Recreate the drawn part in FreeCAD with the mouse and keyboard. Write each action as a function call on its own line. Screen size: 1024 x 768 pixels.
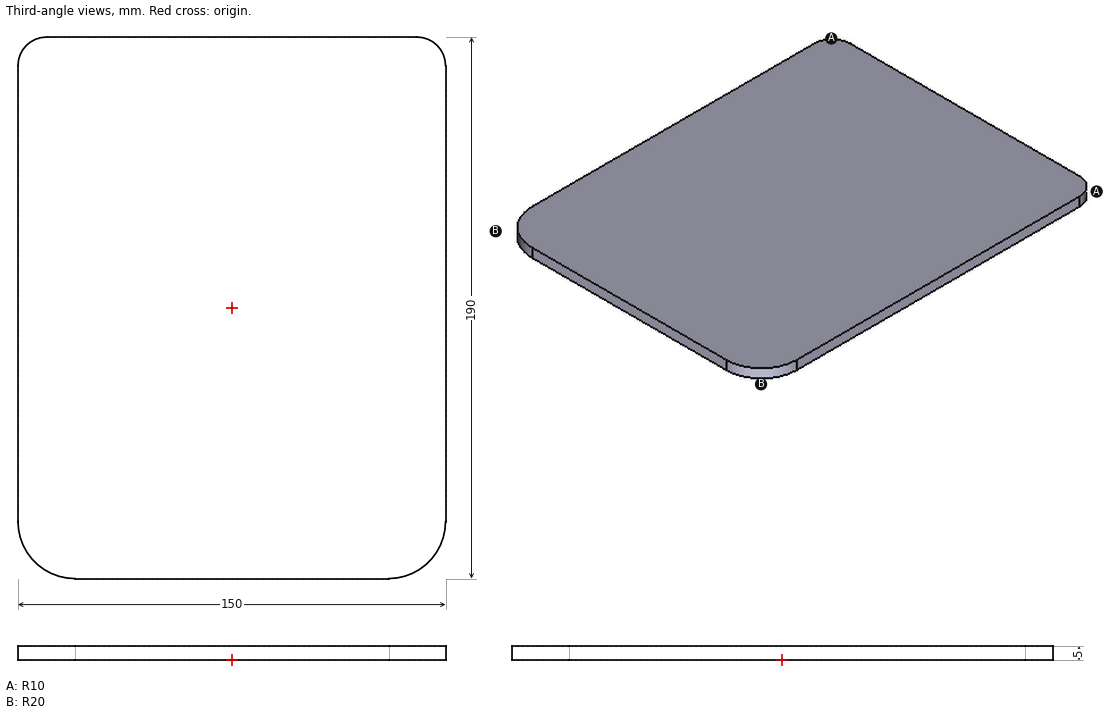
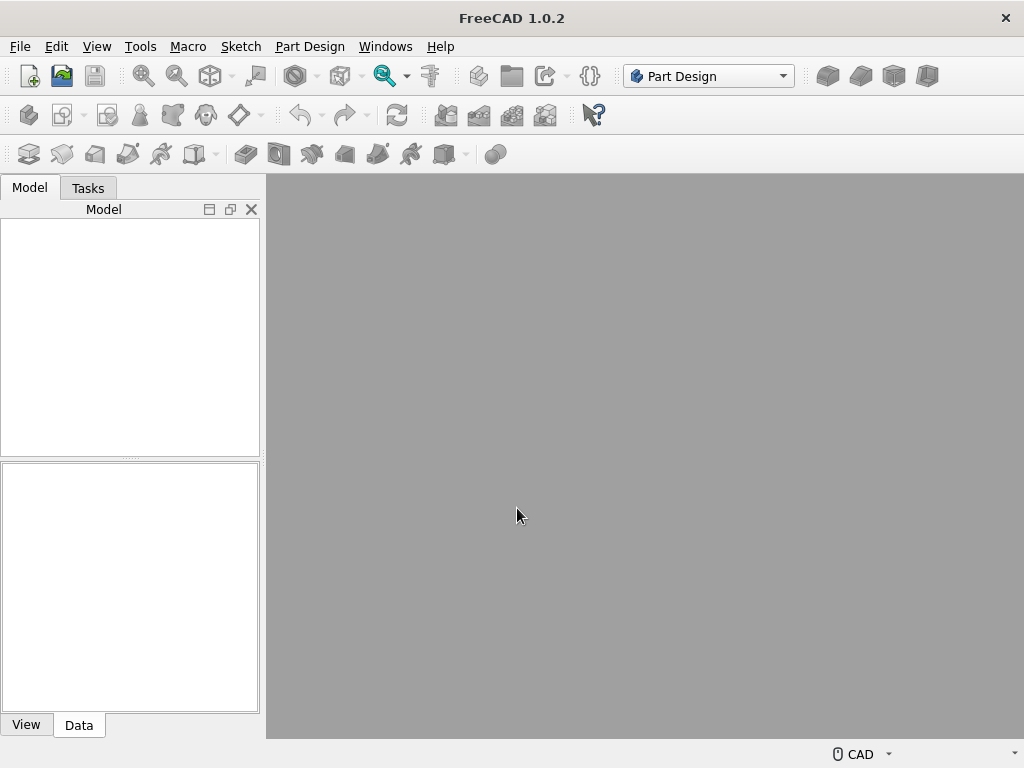
click(29, 76)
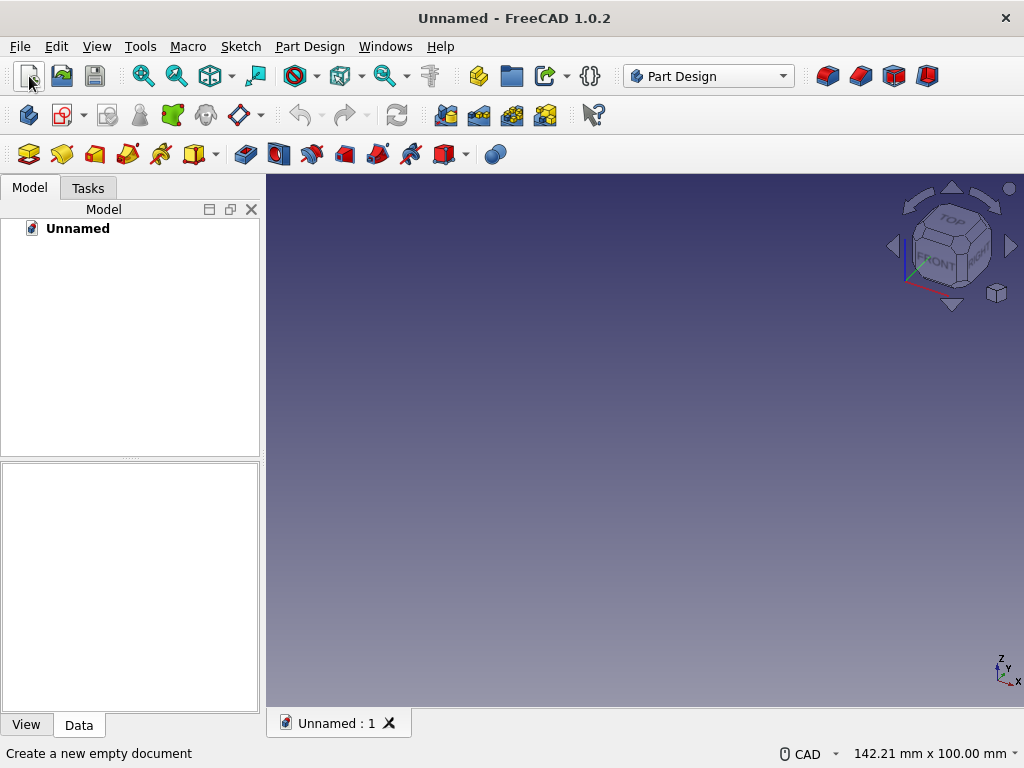
click(62, 116)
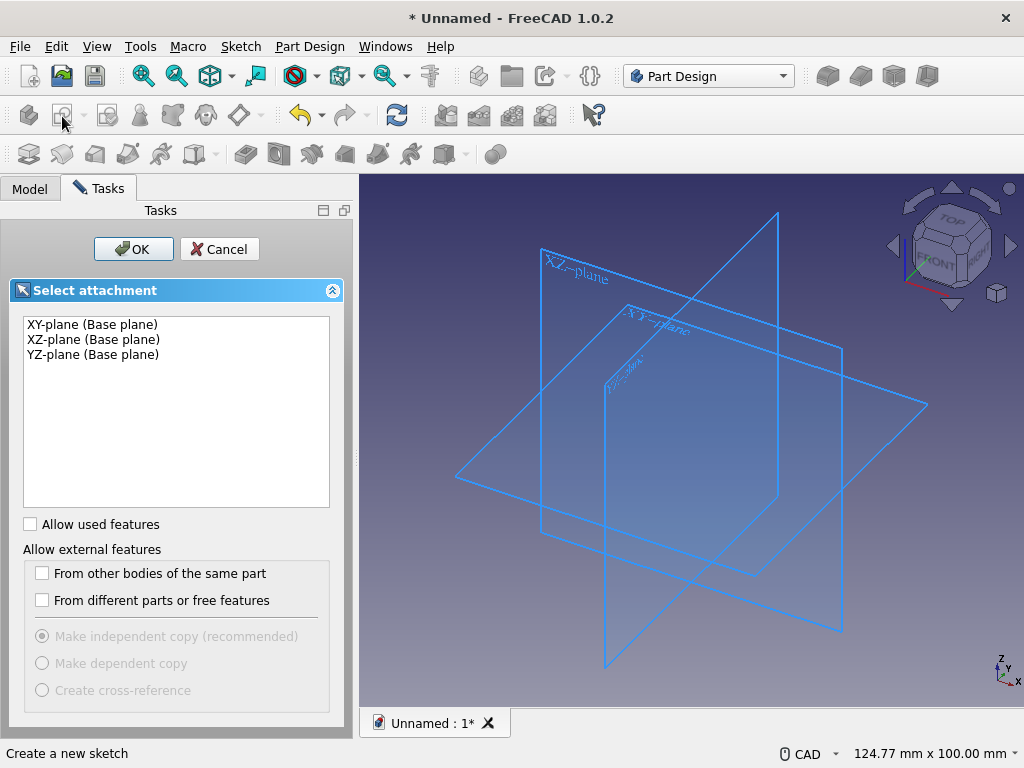
click(84, 324)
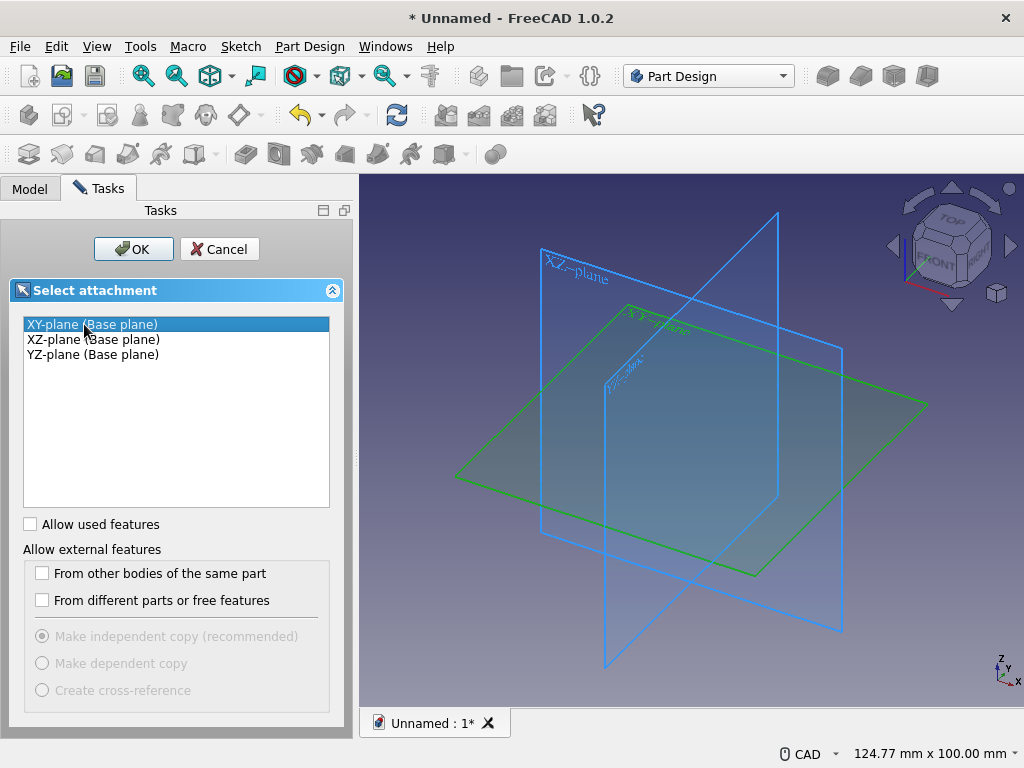
click(134, 249)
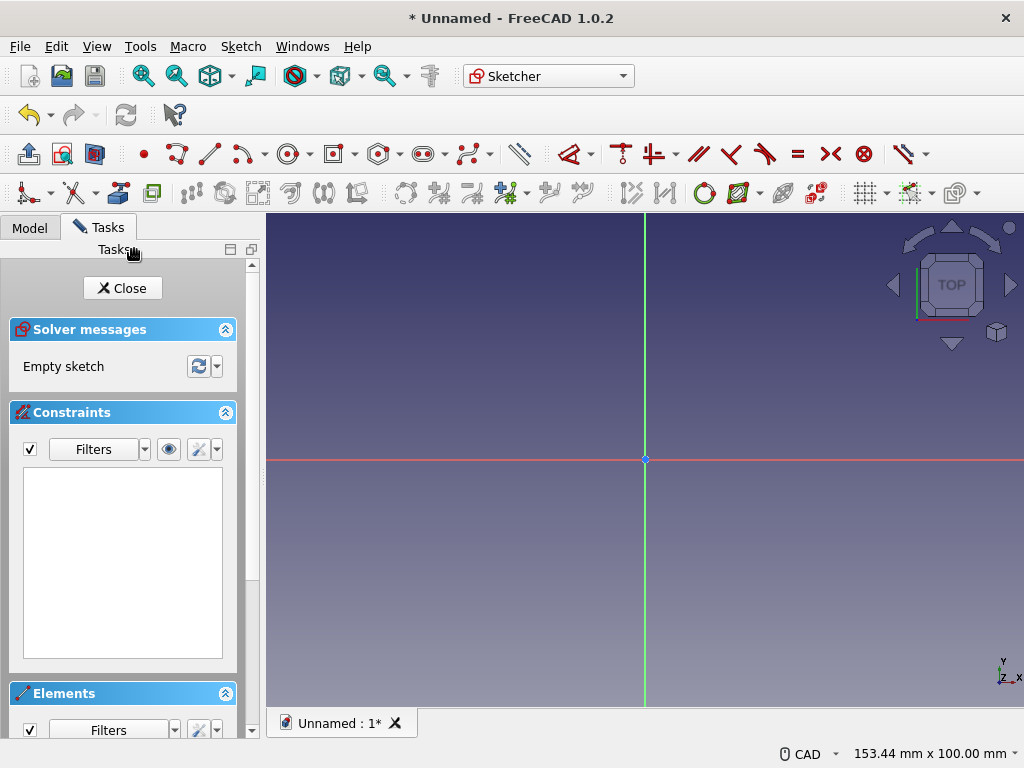
scroll(547, 460, down, 6)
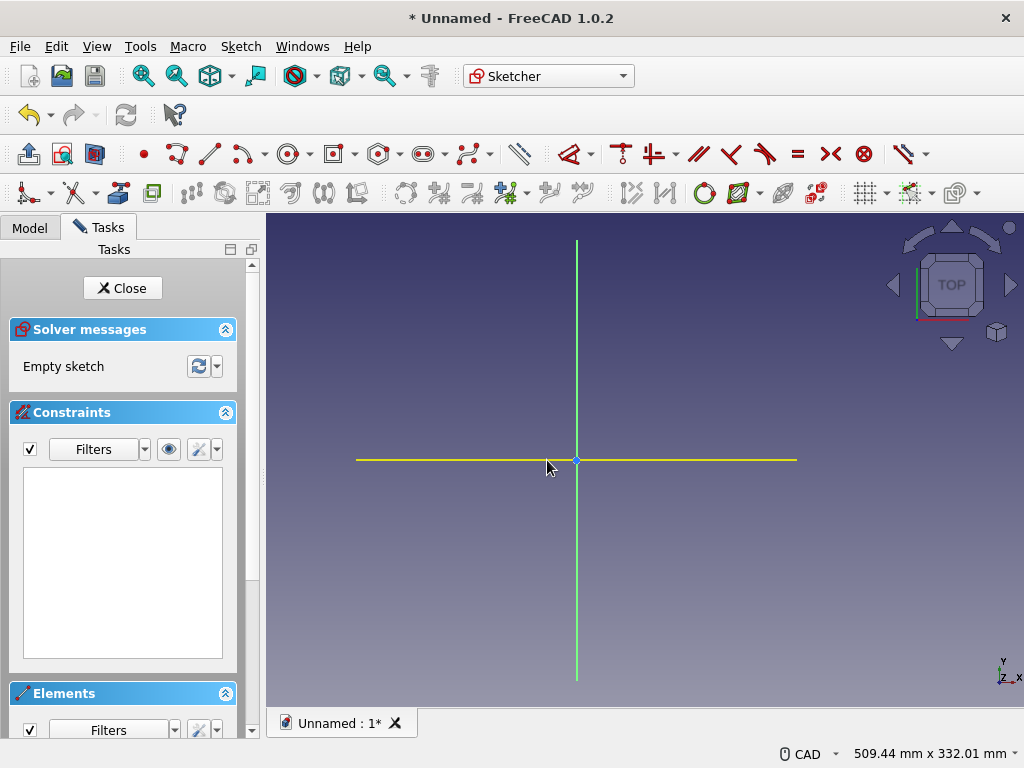
click(332, 154)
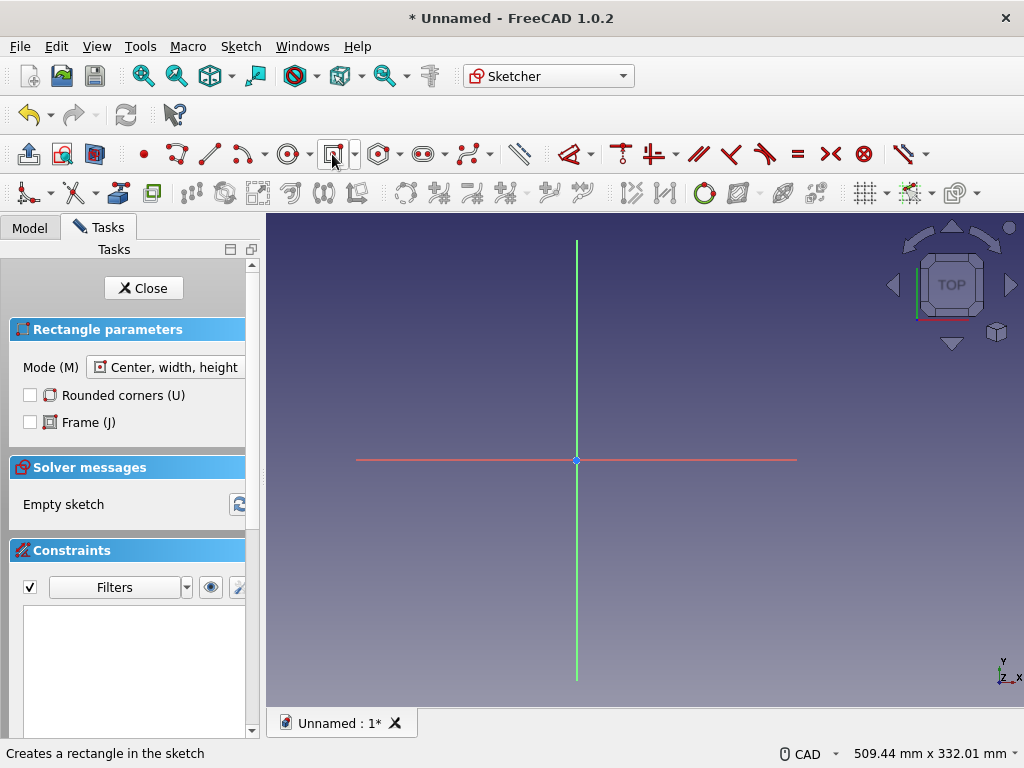
click(577, 460)
click(688, 319)
key(Escape)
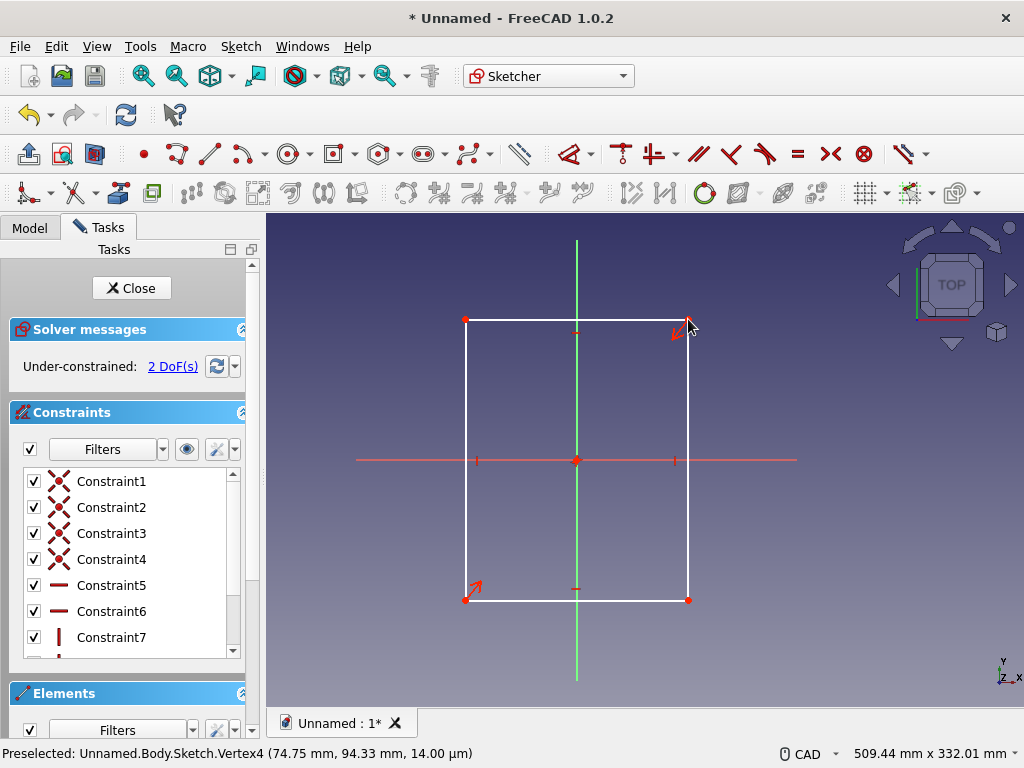
click(568, 154)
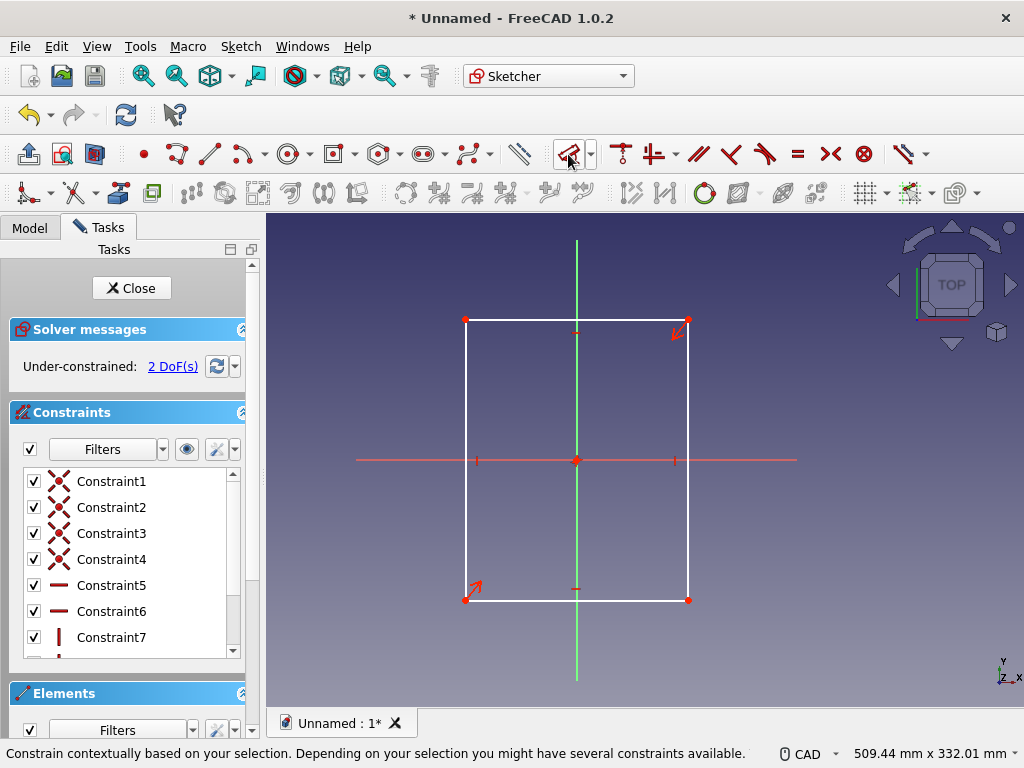
click(532, 601)
click(526, 635)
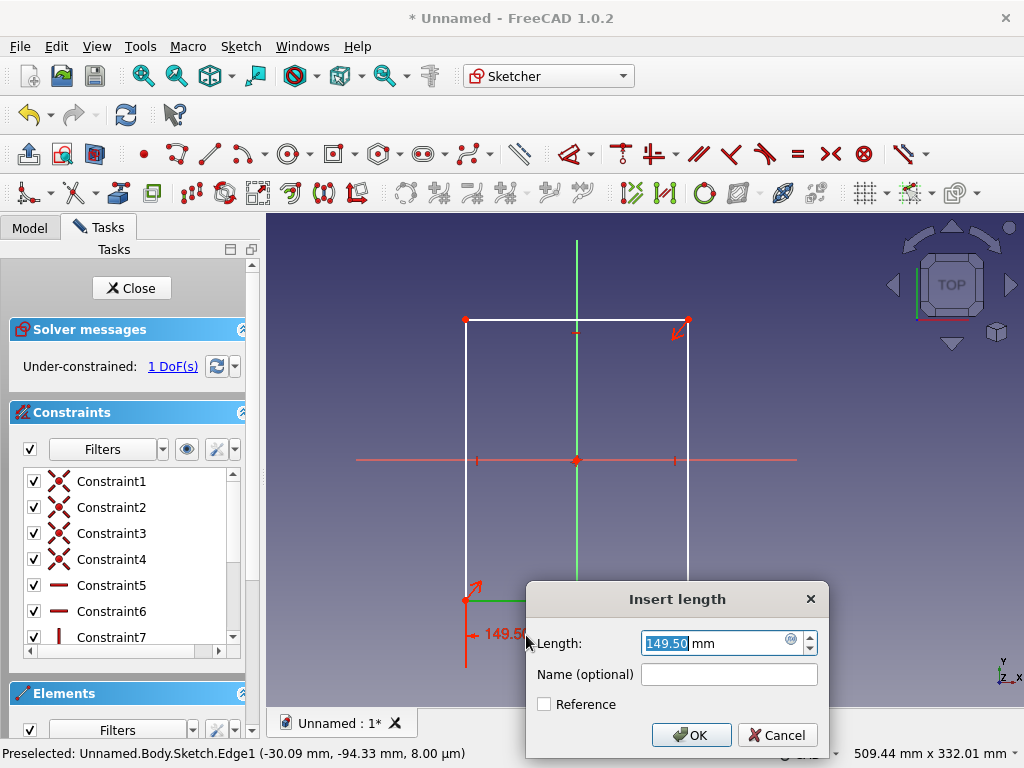
text(150)
key(Return)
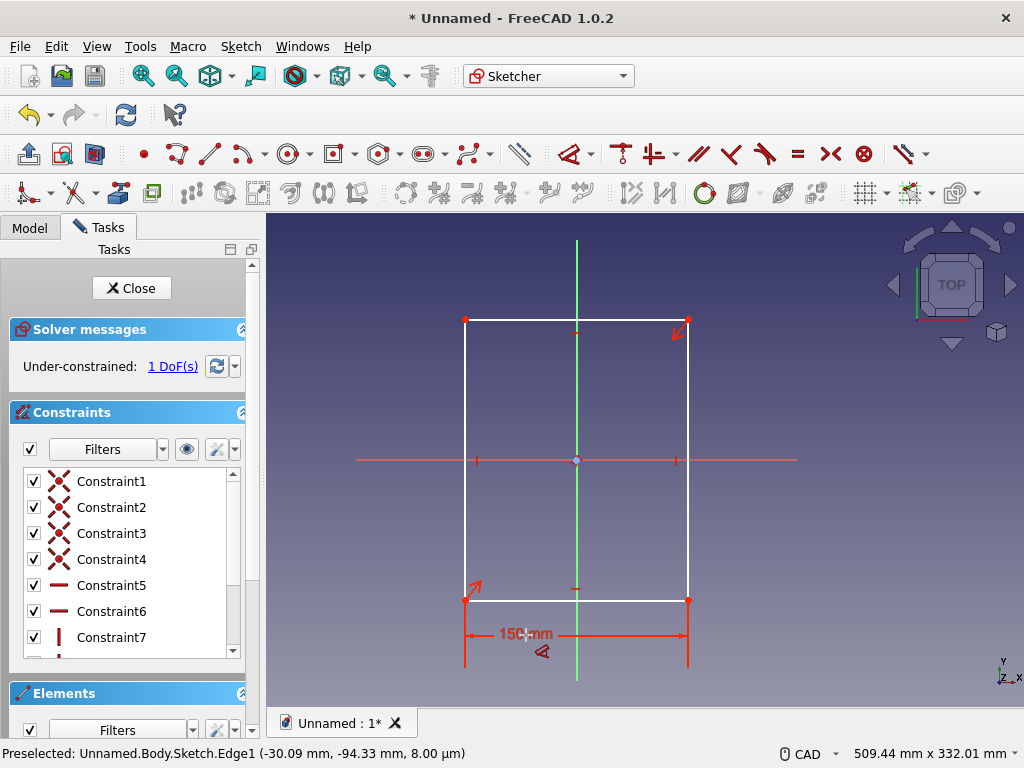
click(688, 516)
click(722, 396)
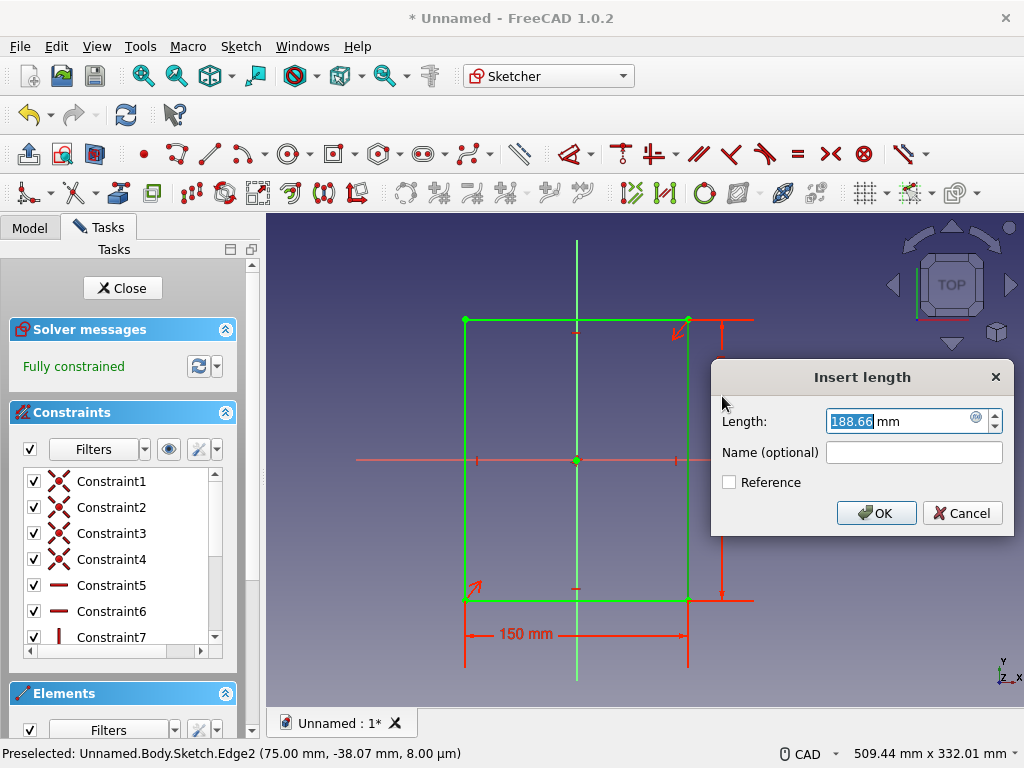
text(190)
key(Return)
key(Escape)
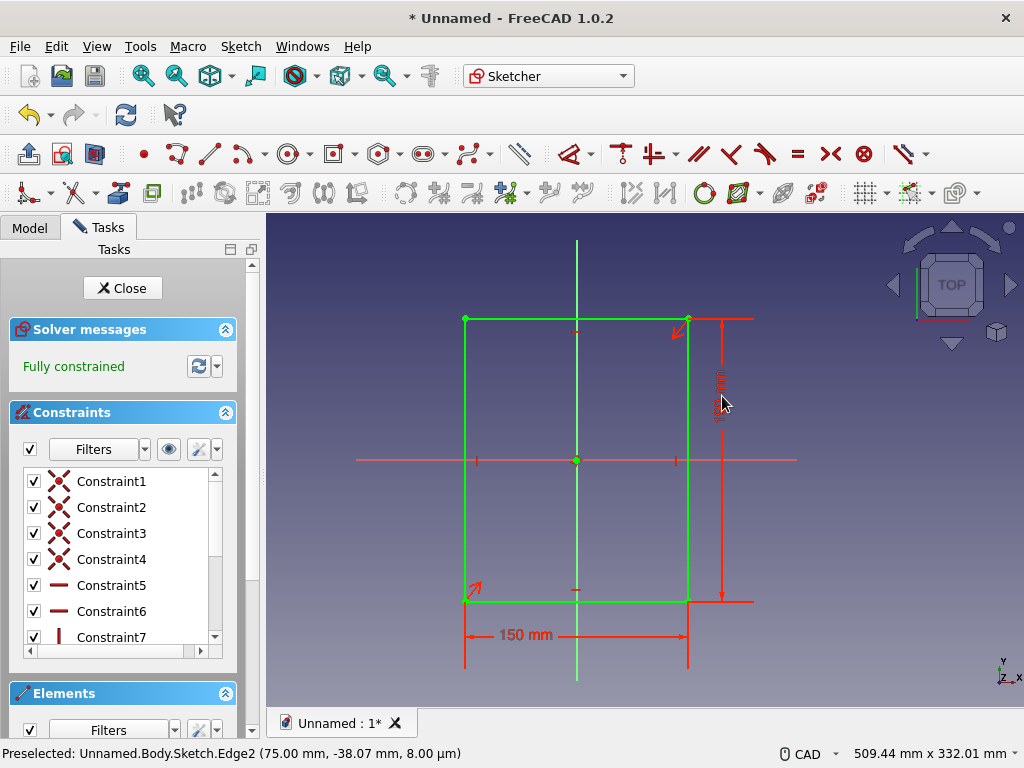
click(123, 288)